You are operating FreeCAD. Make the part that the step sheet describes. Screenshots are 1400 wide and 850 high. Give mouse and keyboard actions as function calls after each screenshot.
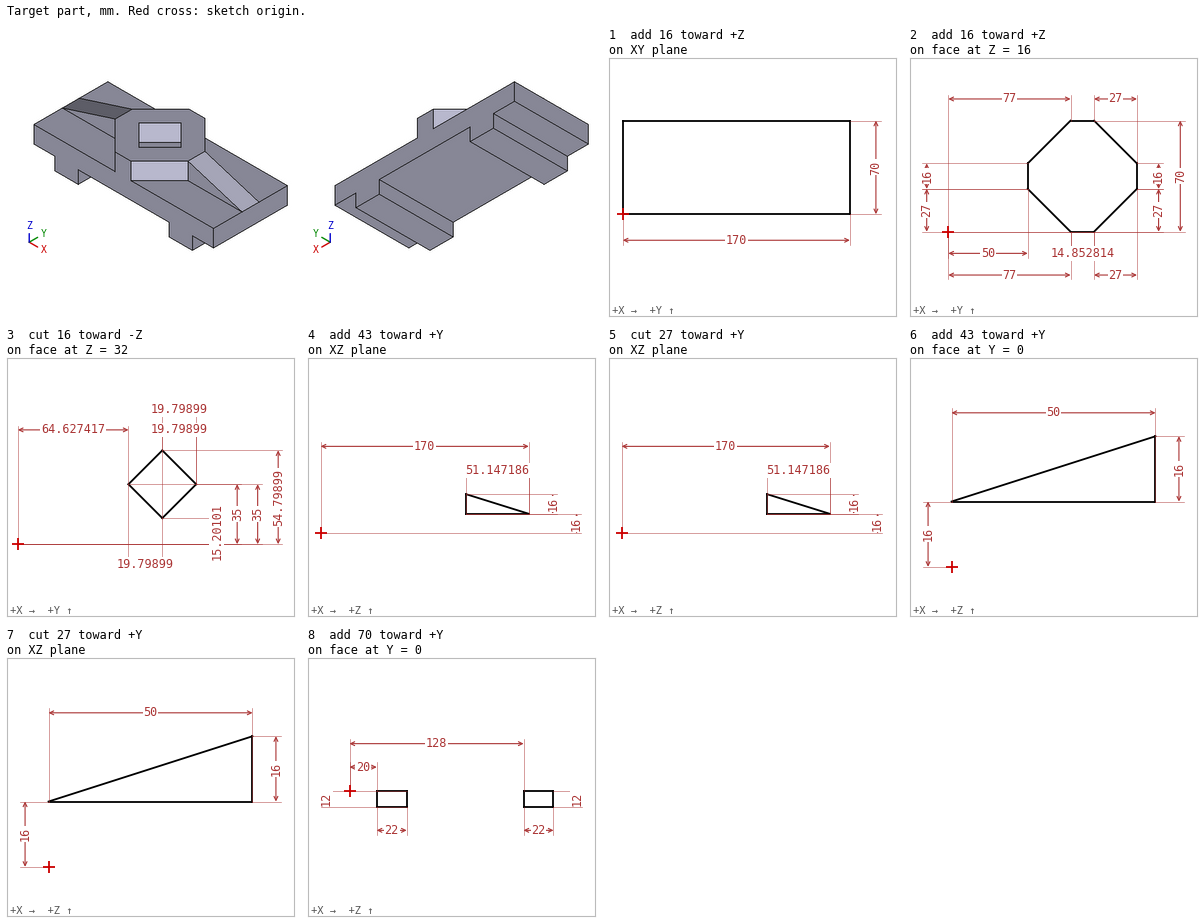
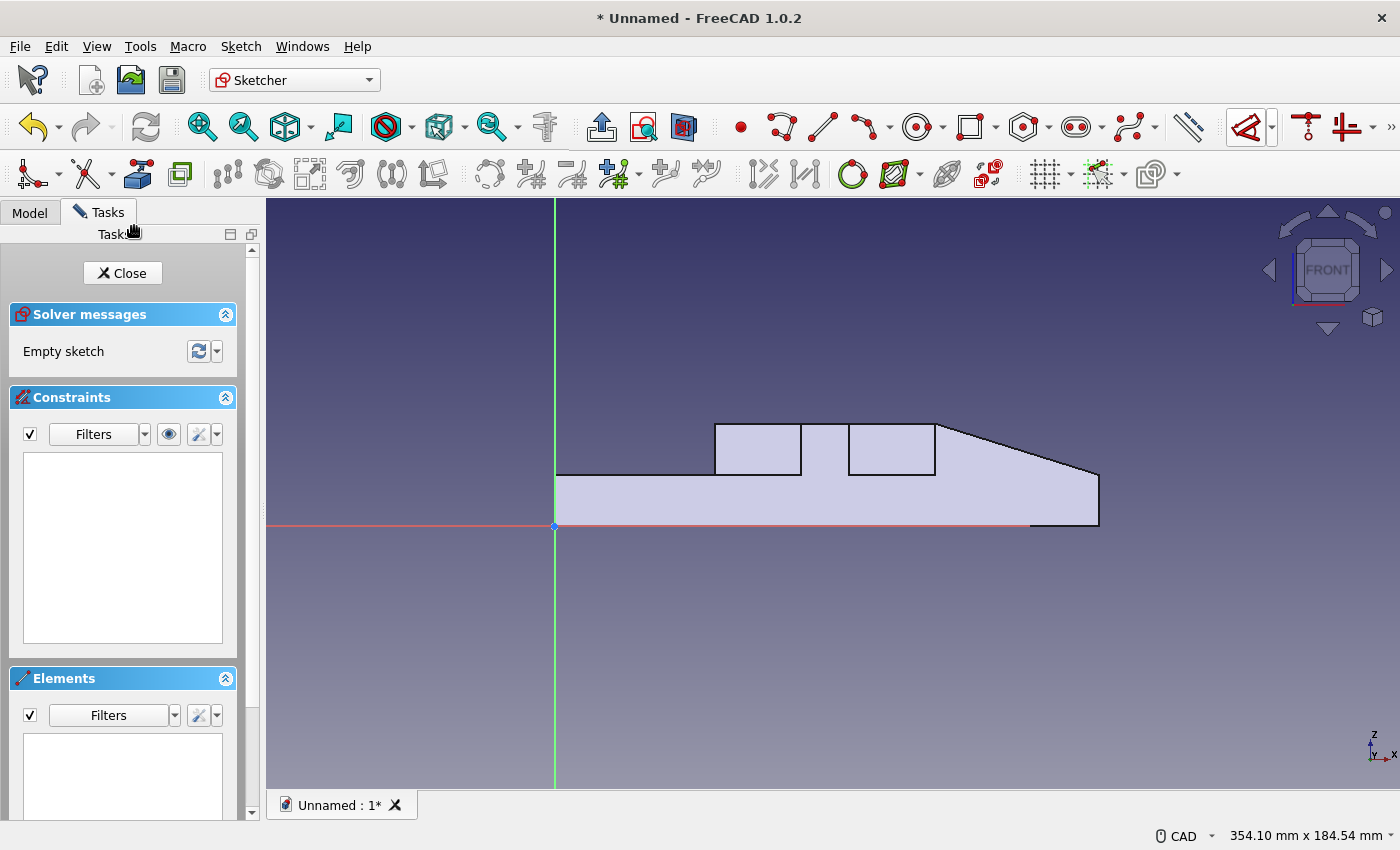
scroll(1100, 435, up, 7)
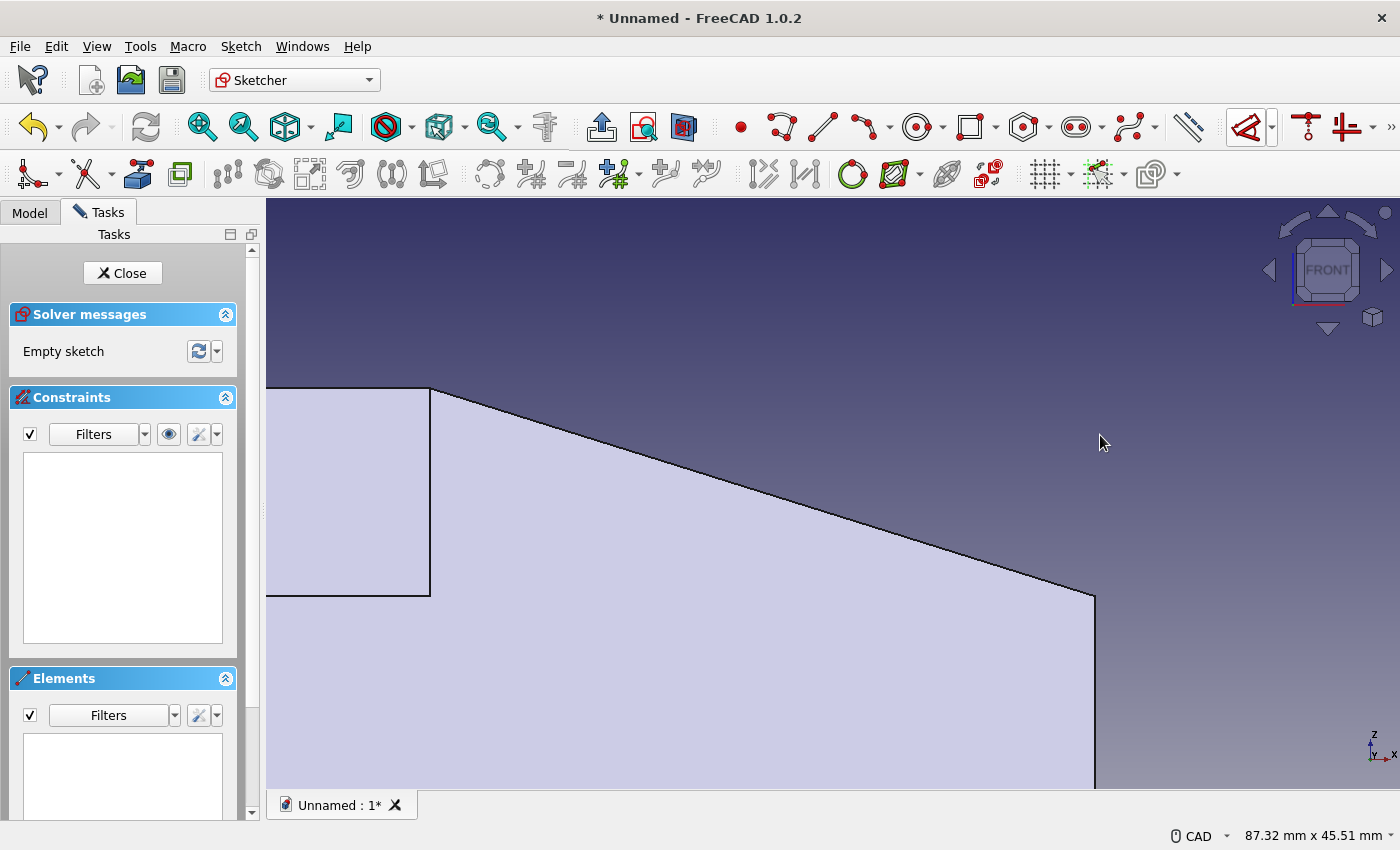
key(g)
key(m)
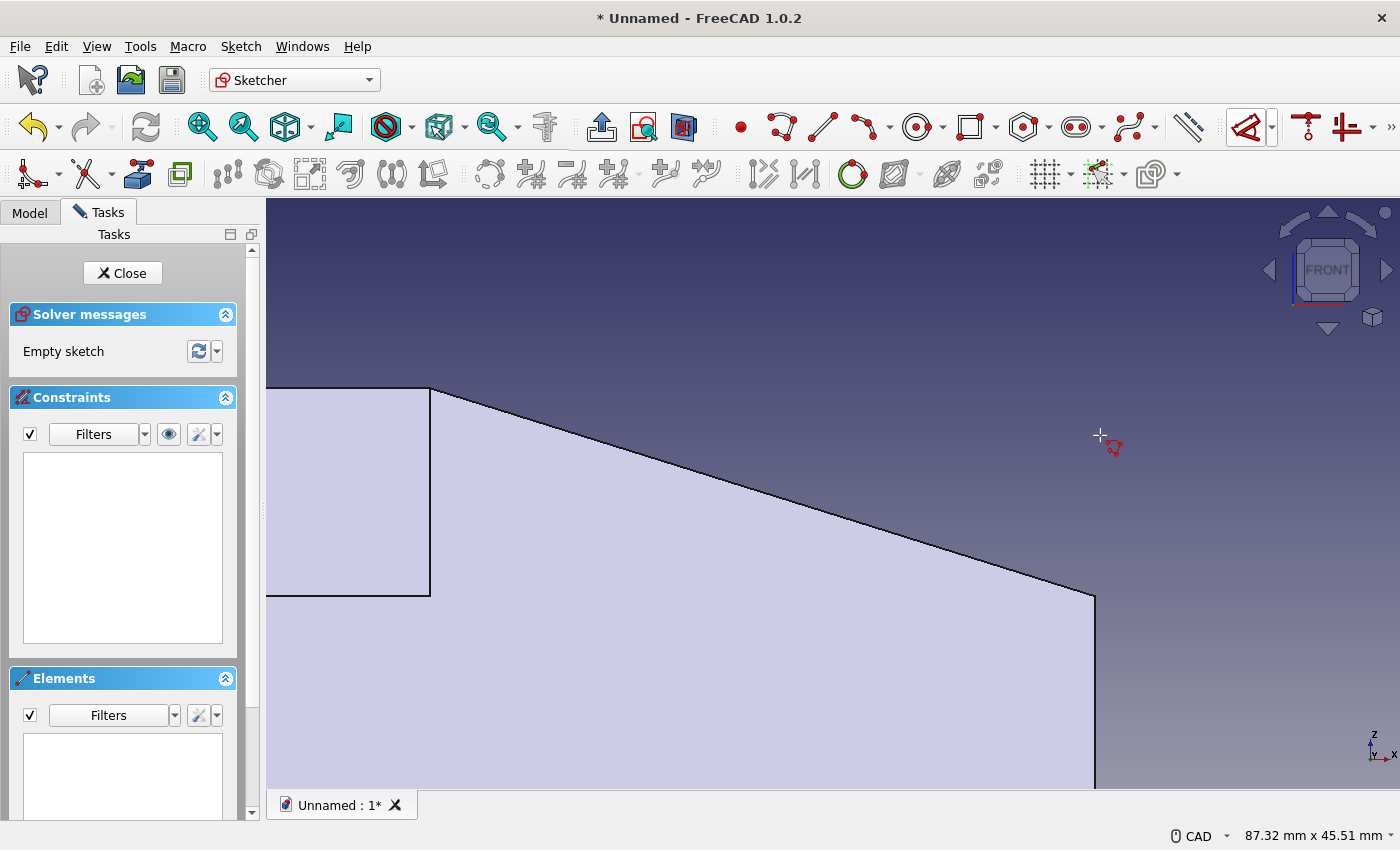
click(430, 596)
click(1095, 596)
click(430, 388)
click(430, 597)
key(Escape)
key(Escape)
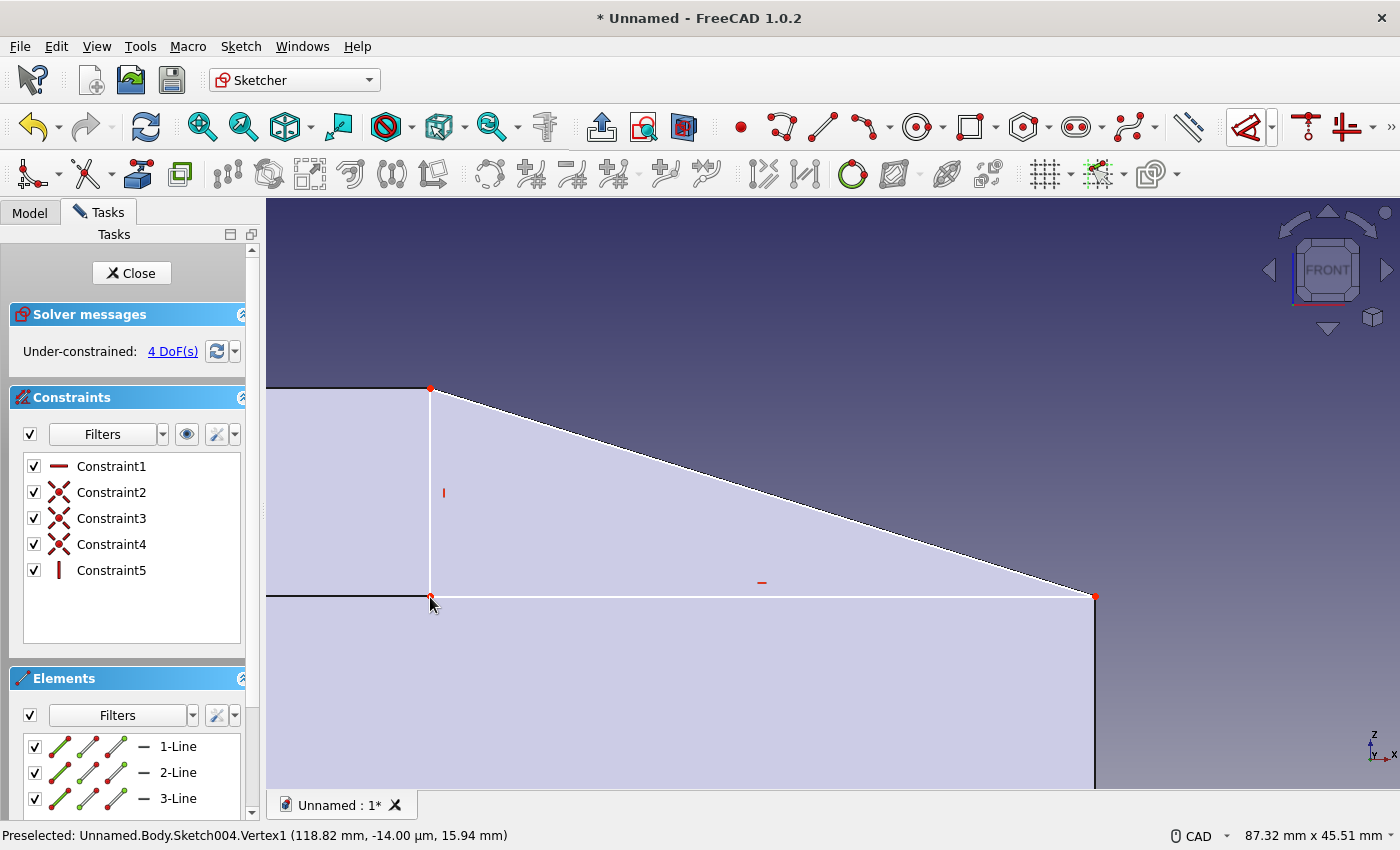
key(d)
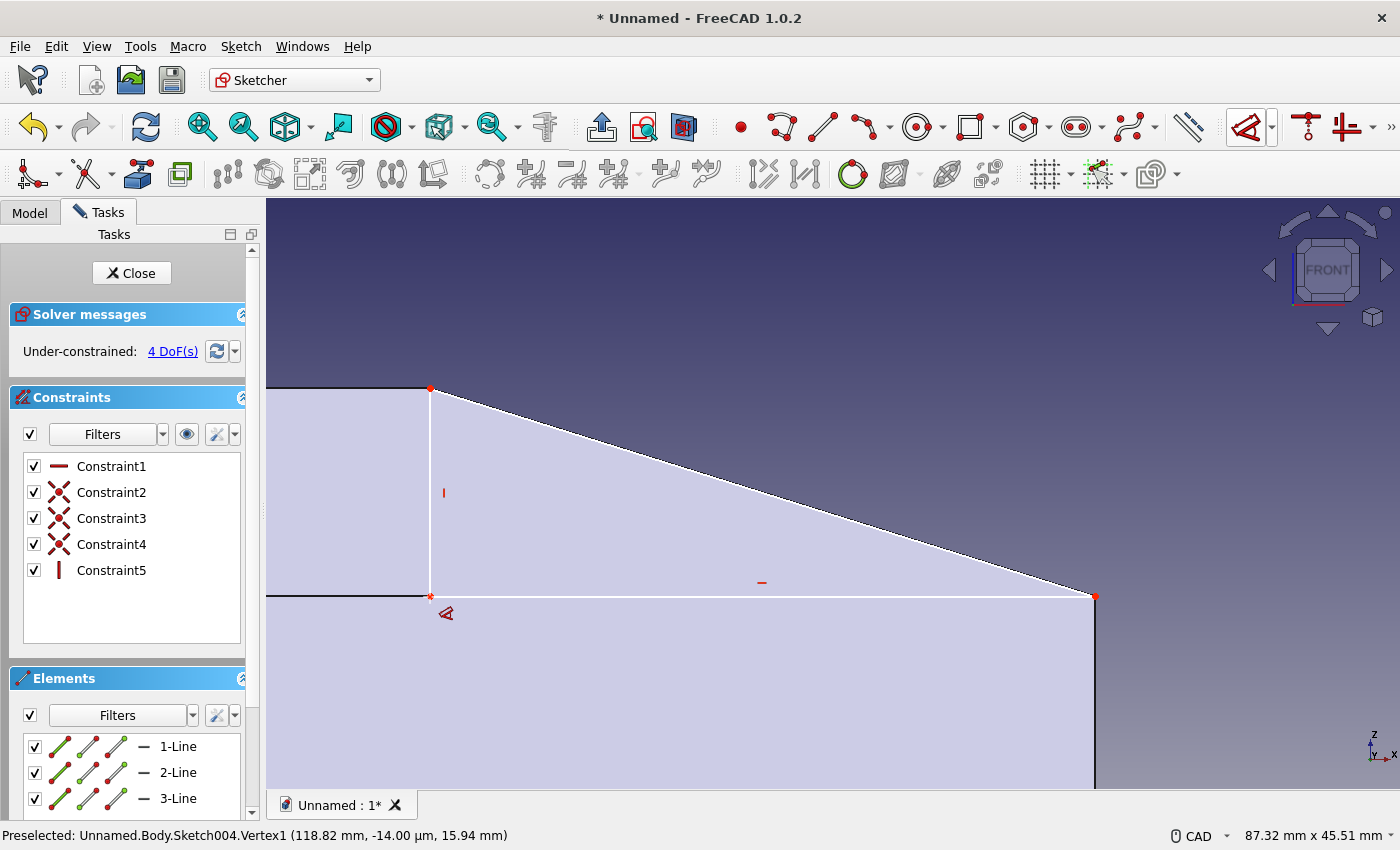
click(430, 451)
click(396, 493)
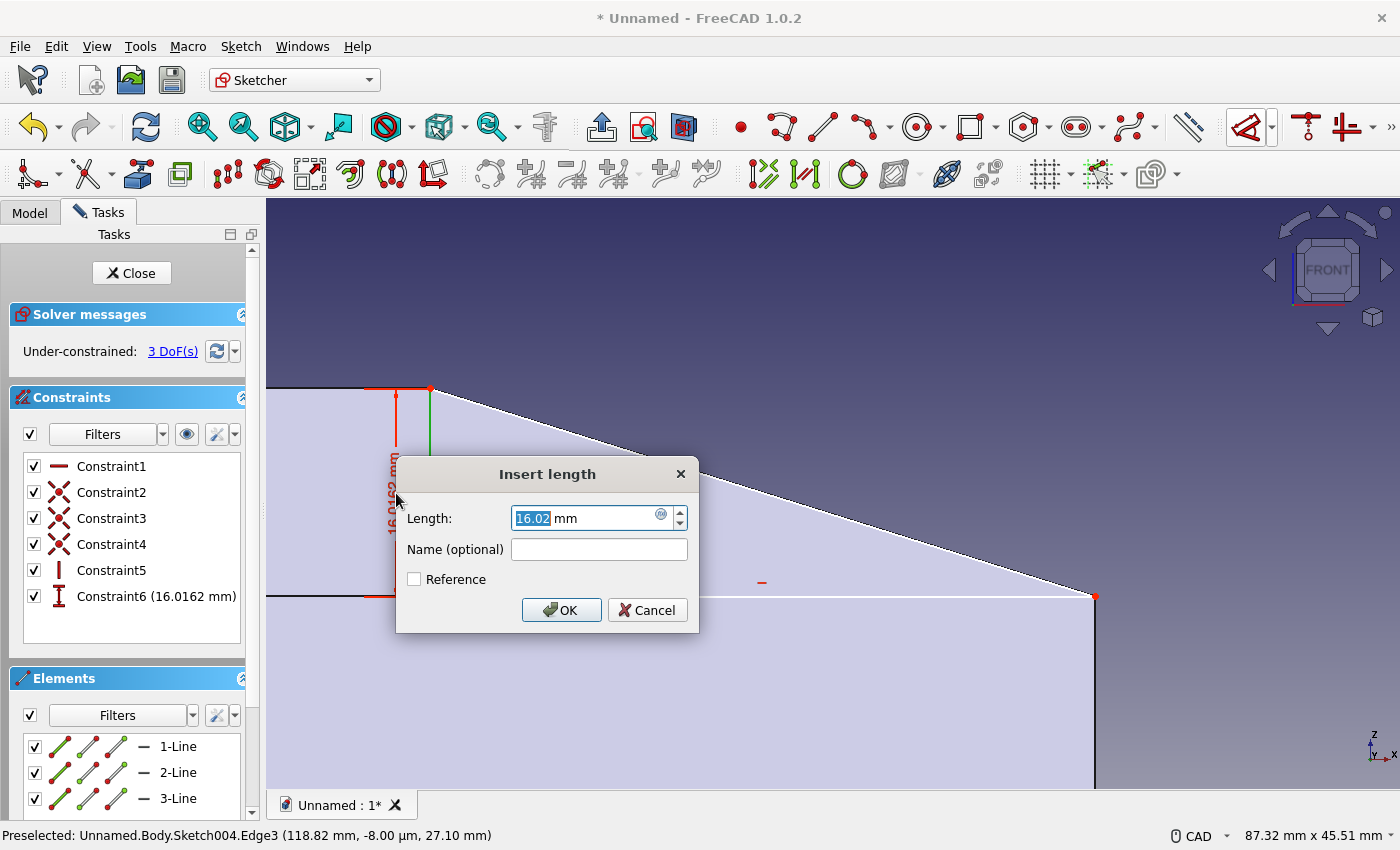
text(16)
key(Return)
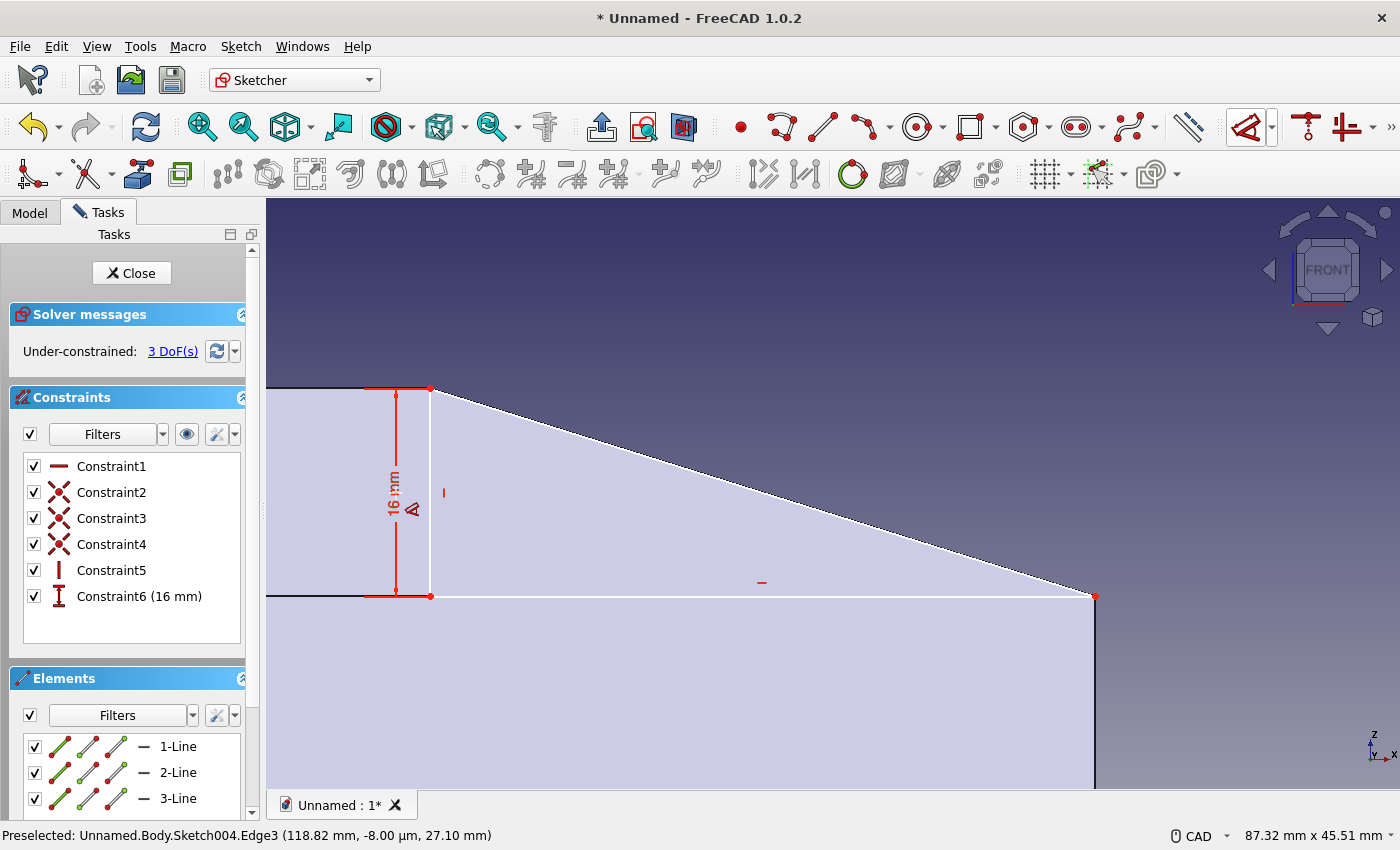
click(430, 597)
click(464, 679)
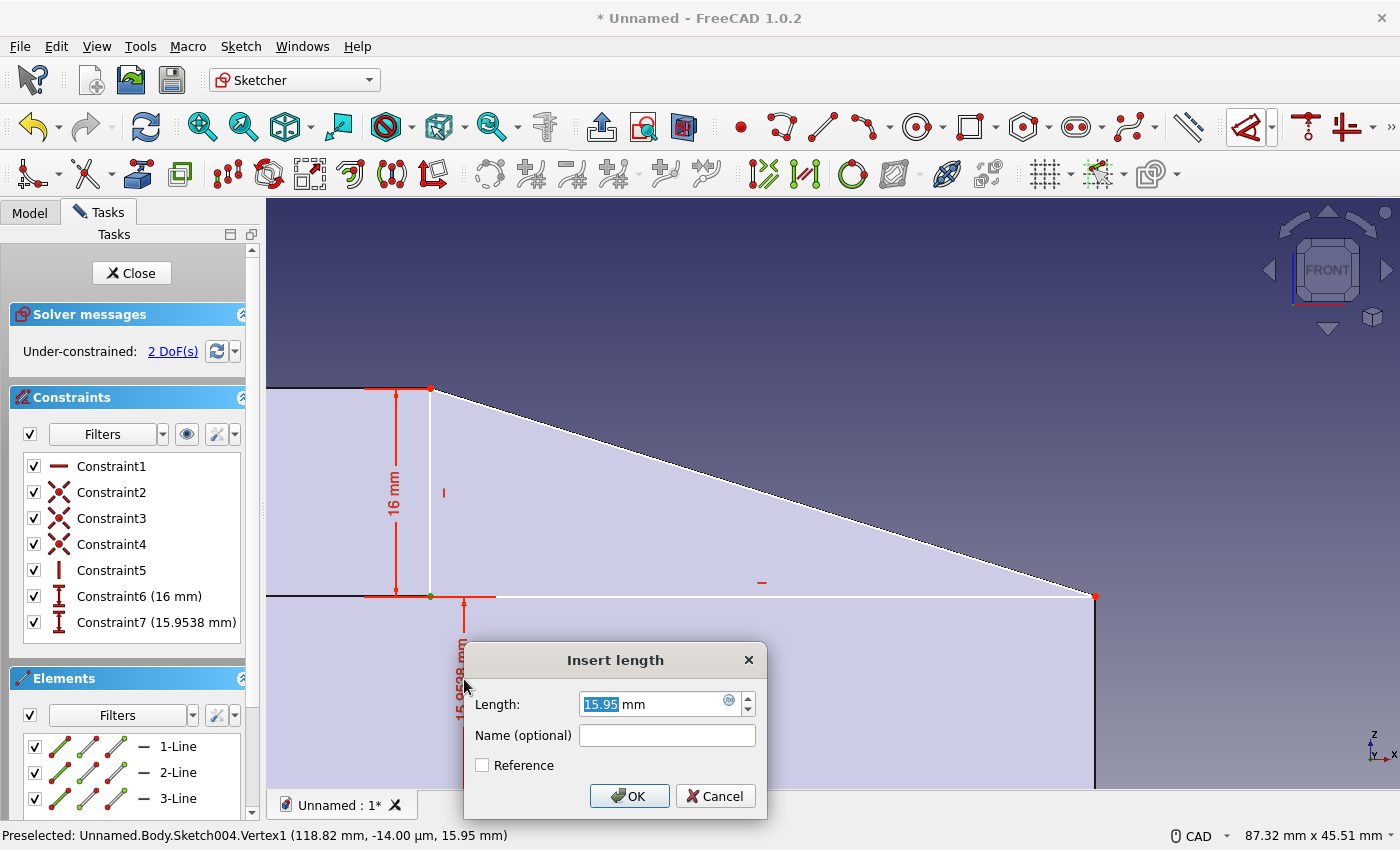
text(16)
key(Return)